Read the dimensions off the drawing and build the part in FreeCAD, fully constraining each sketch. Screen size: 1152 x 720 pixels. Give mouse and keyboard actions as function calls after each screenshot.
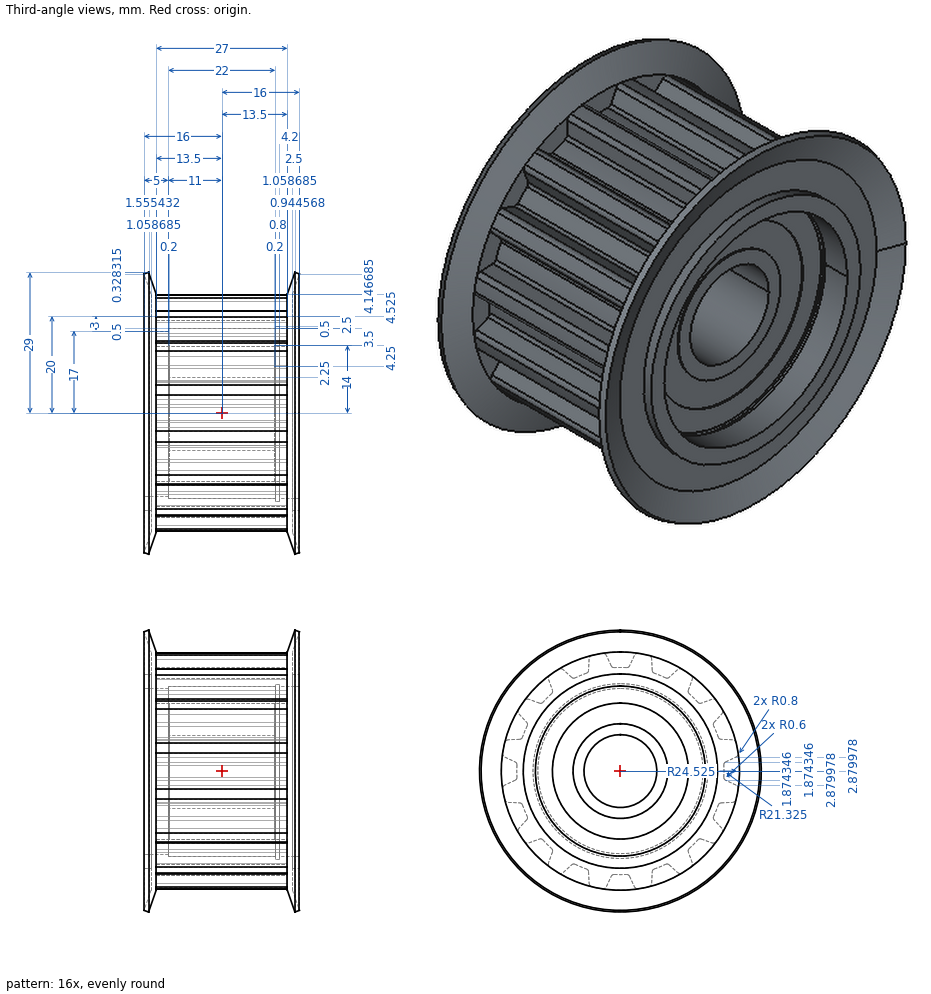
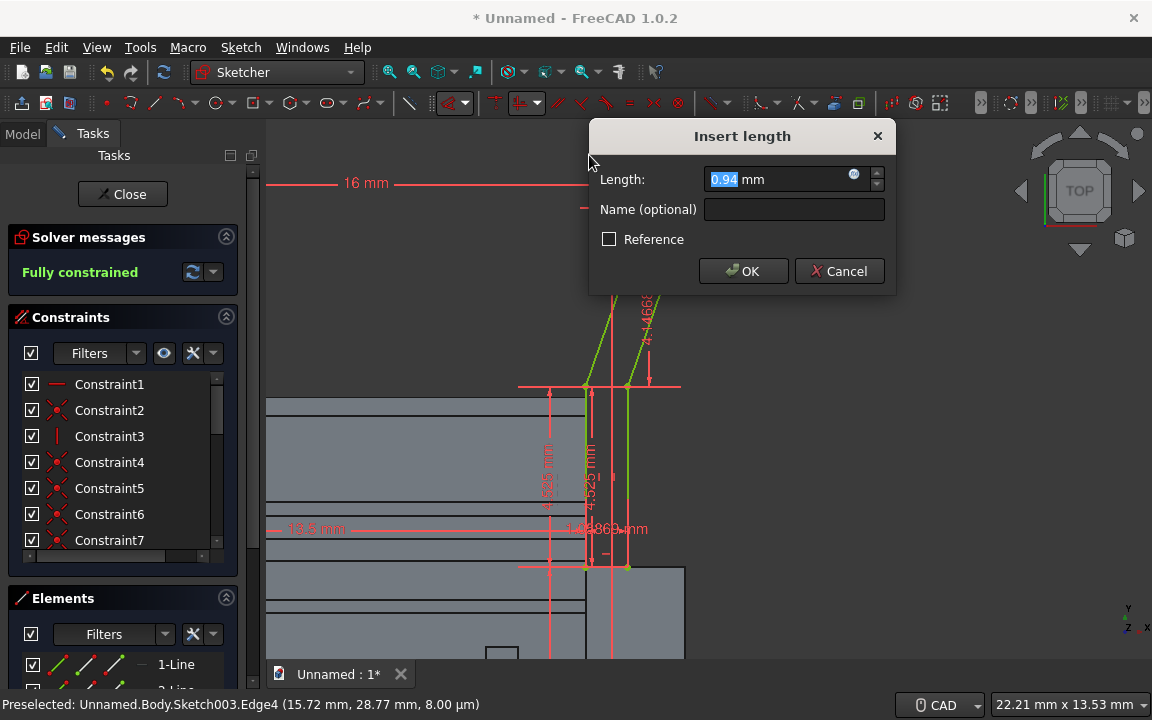
text(0.944568)
key(Return)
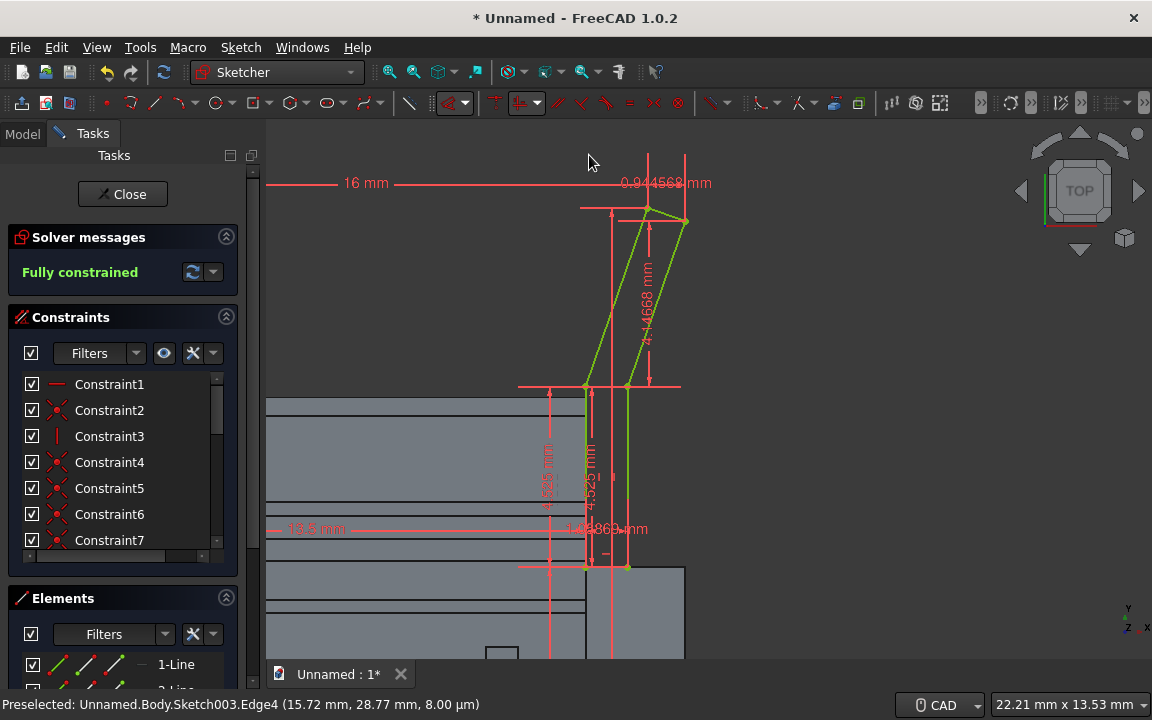
click(123, 194)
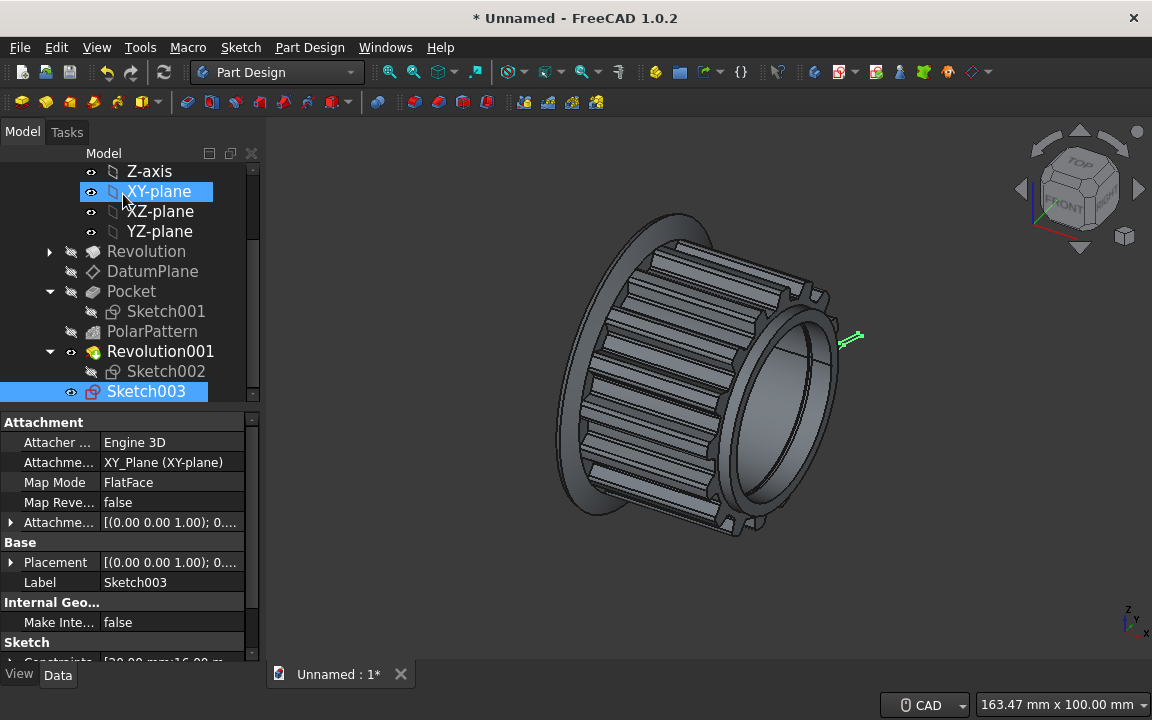
click(46, 102)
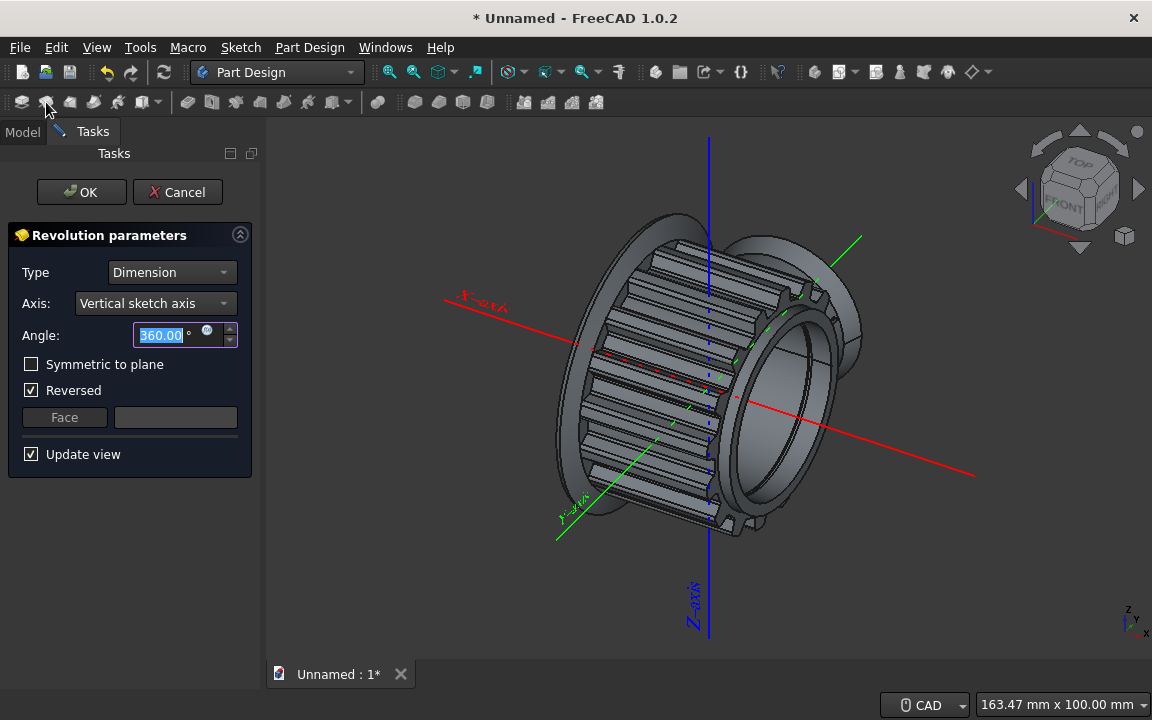
click(156, 304)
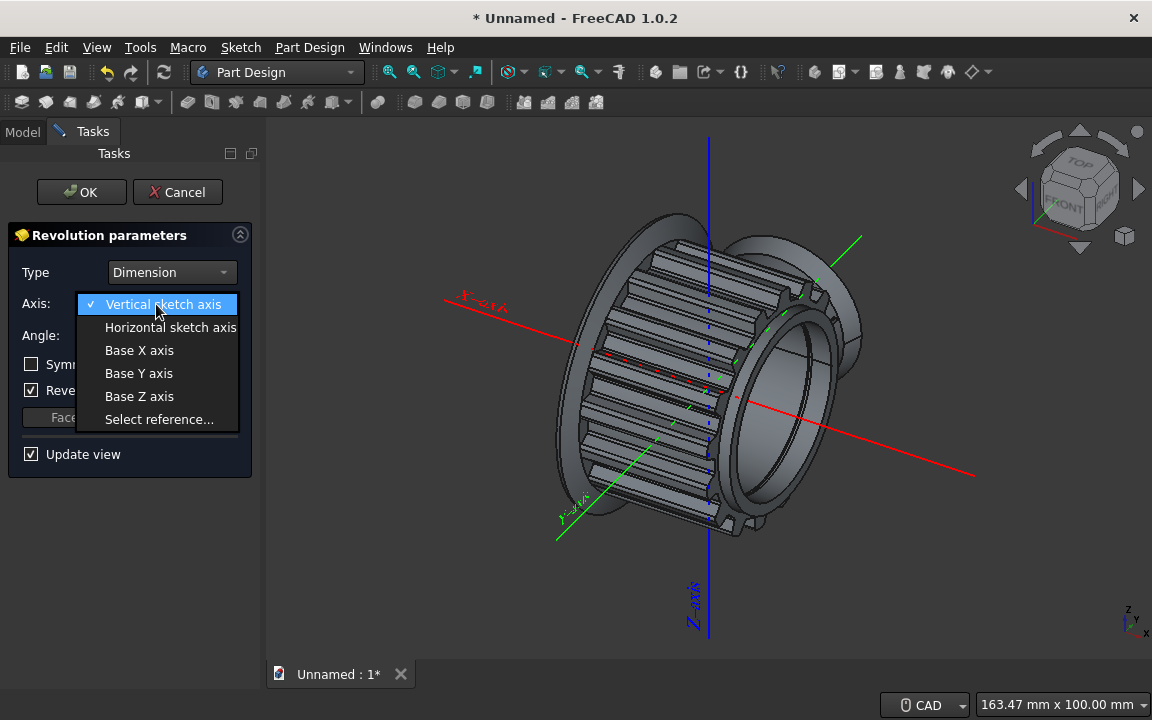
click(156, 328)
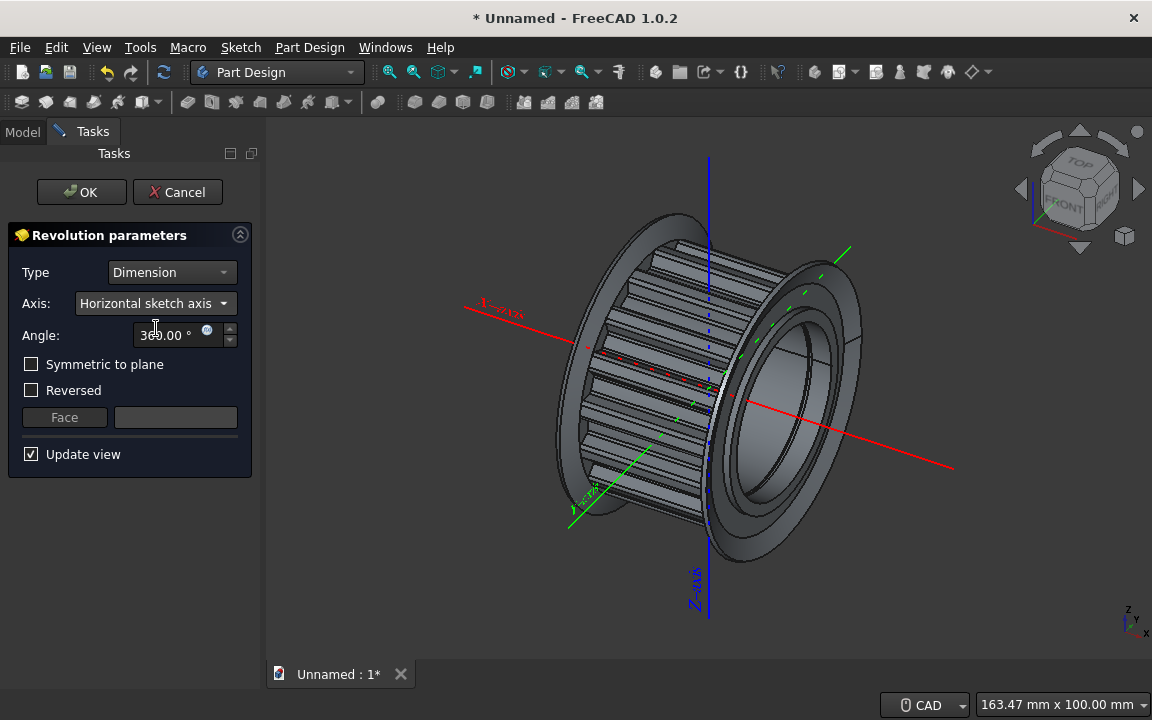
click(82, 192)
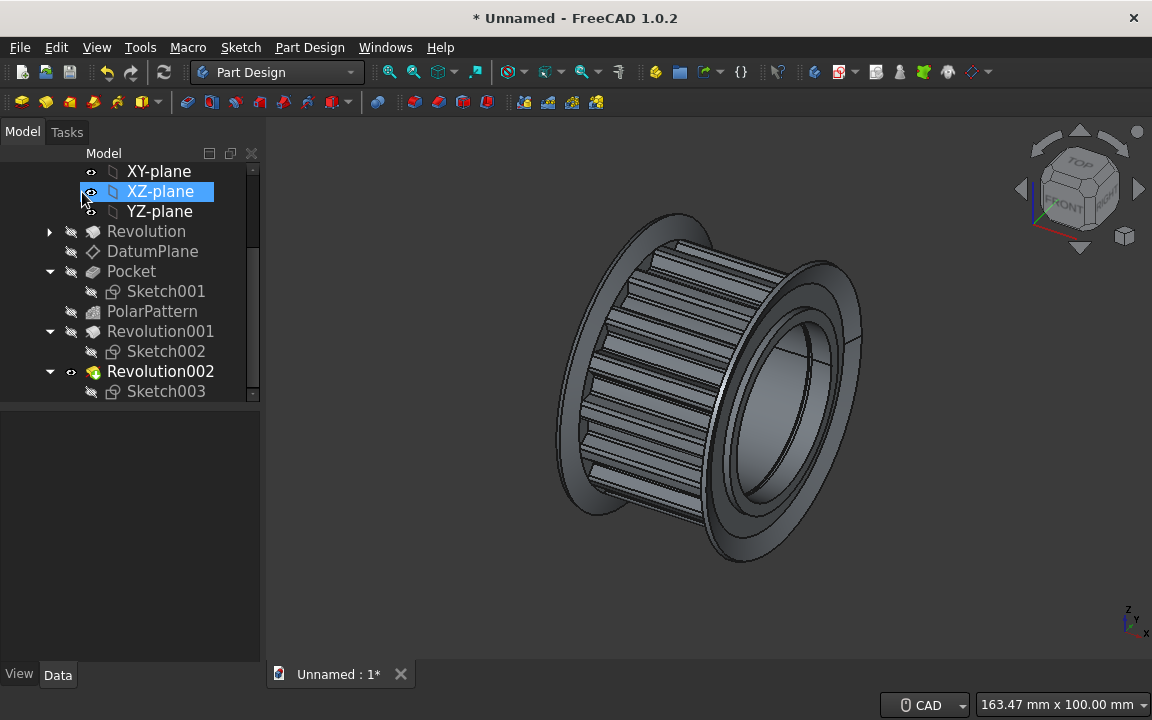
click(816, 72)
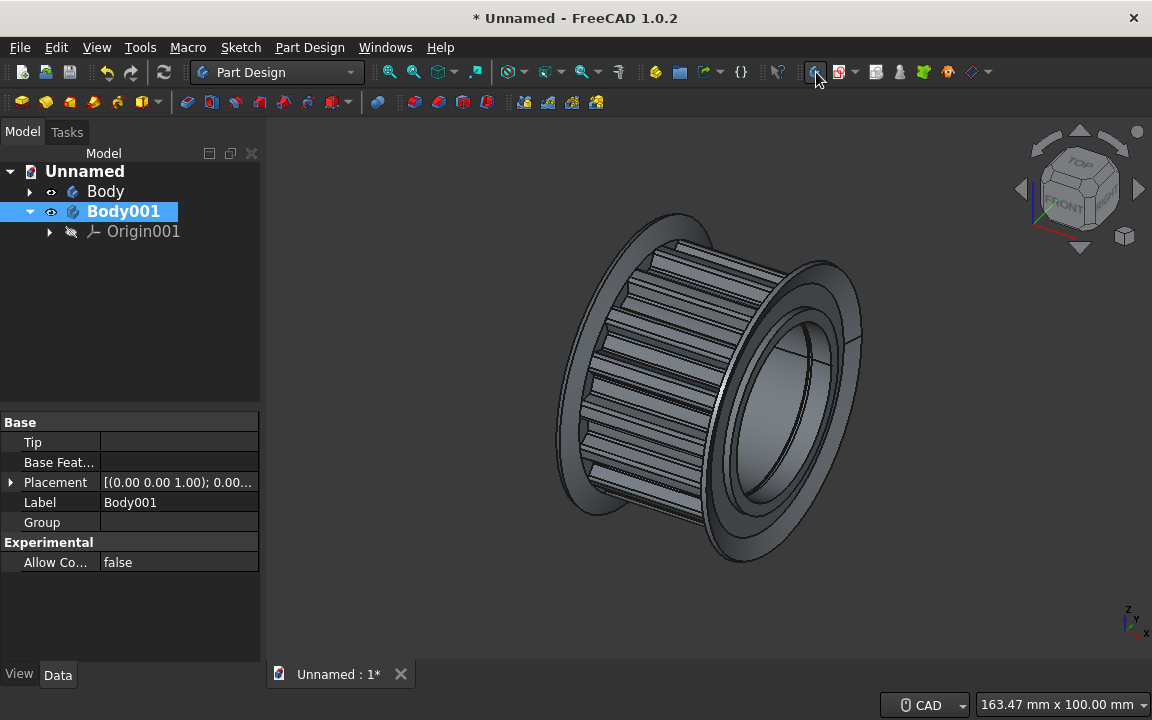
click(306, 619)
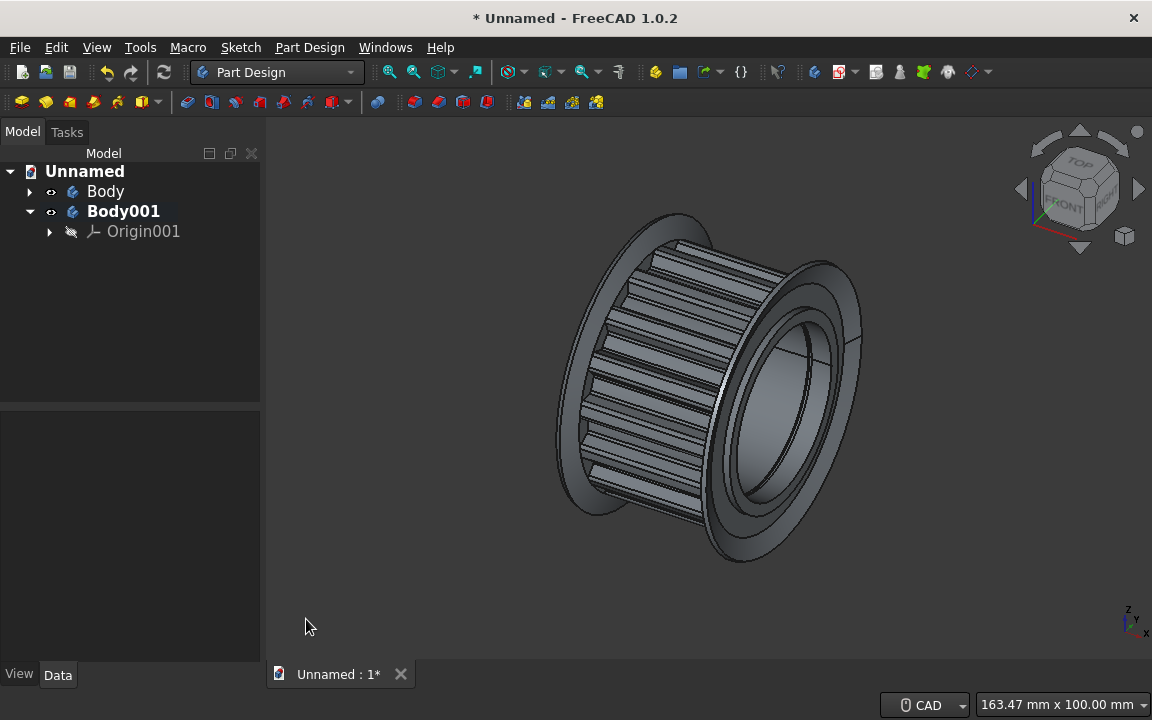
click(840, 72)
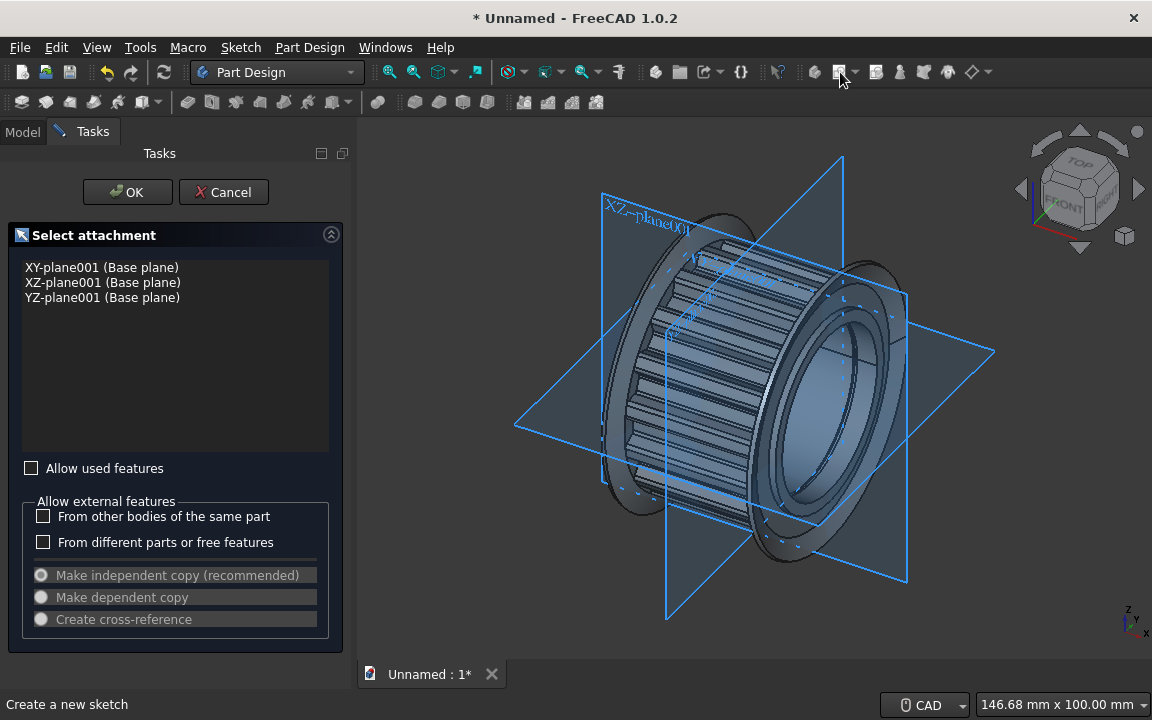
click(82, 268)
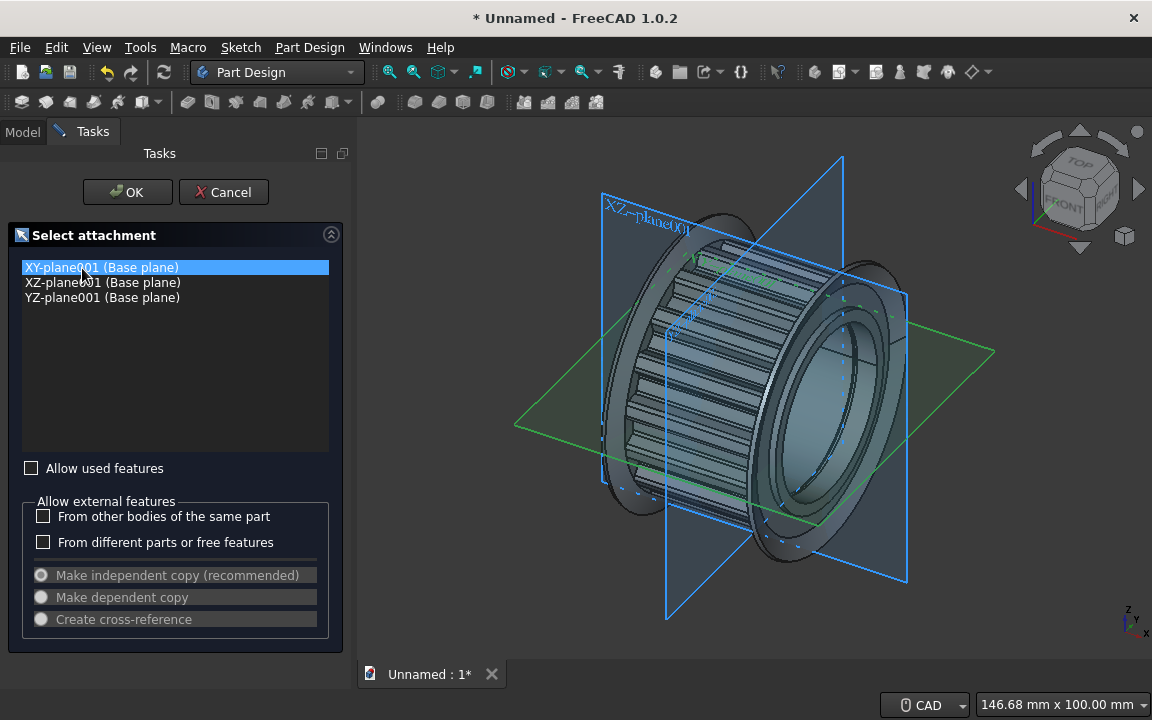
click(128, 192)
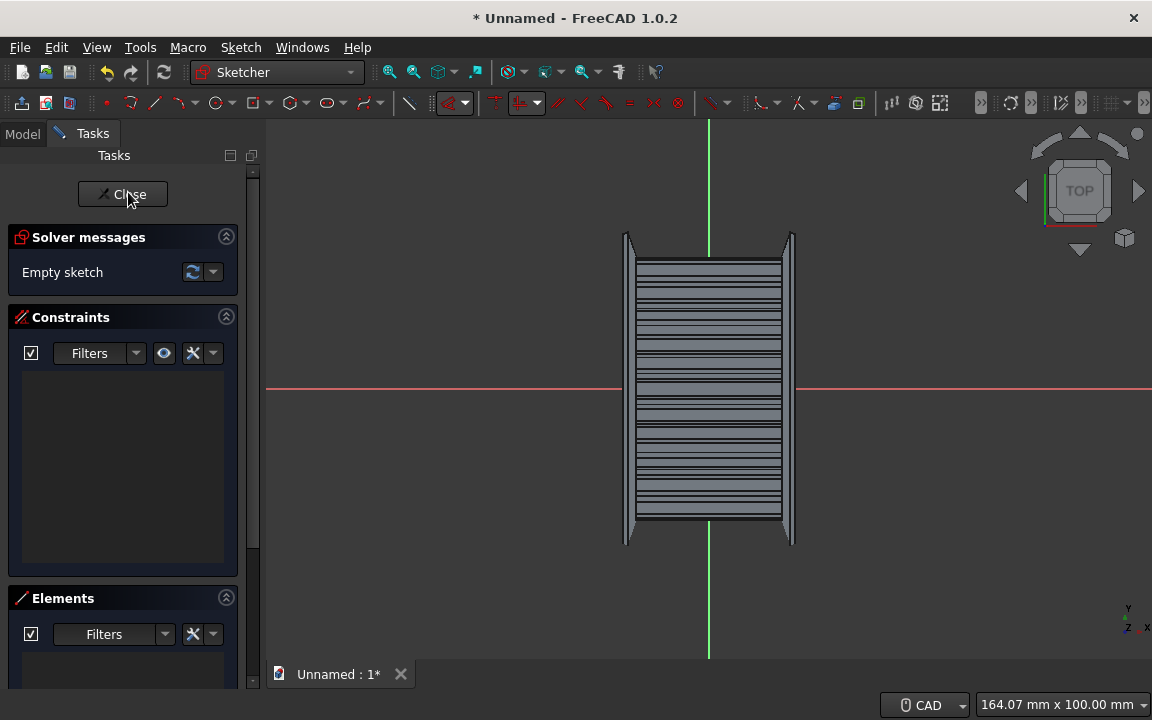
scroll(739, 321, up, 6)